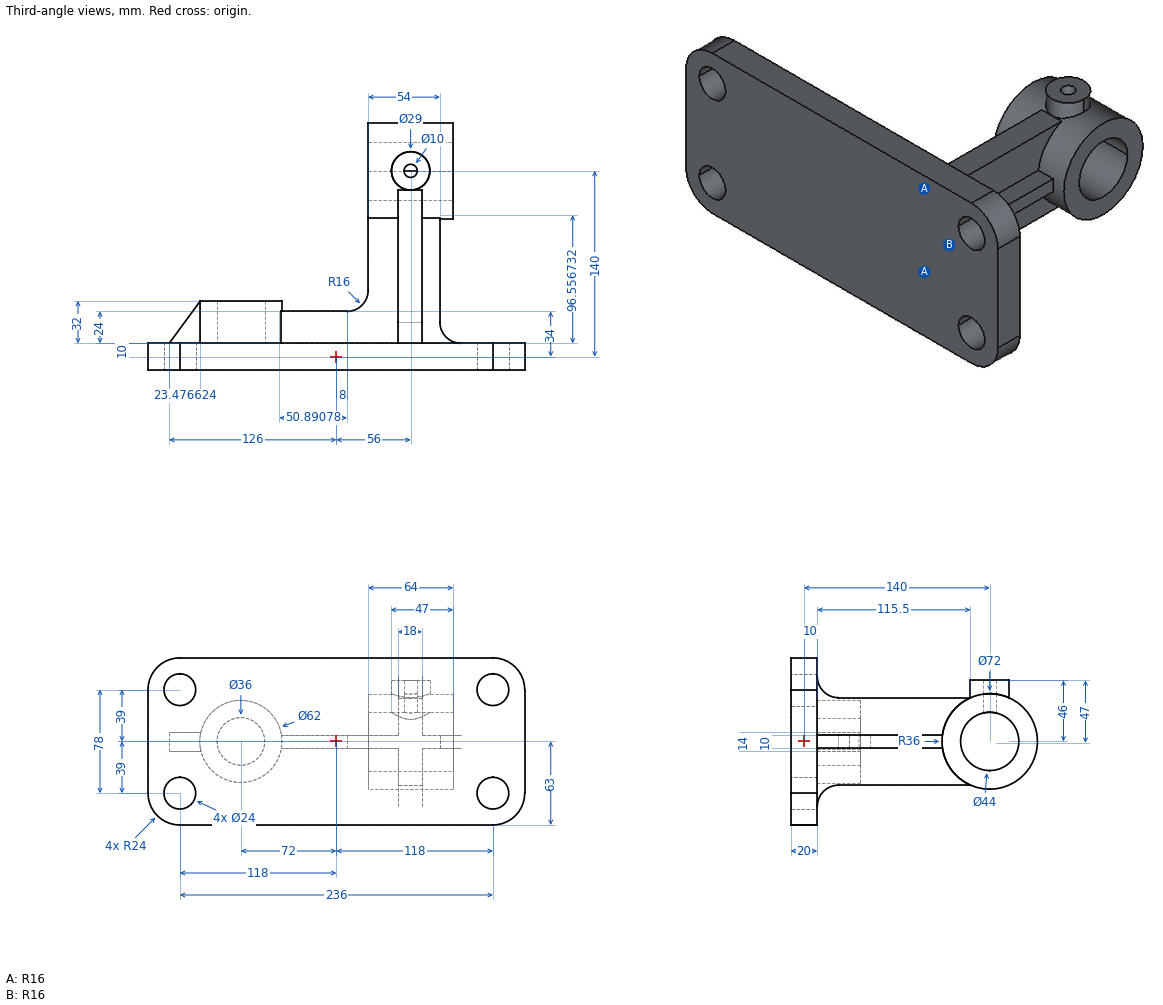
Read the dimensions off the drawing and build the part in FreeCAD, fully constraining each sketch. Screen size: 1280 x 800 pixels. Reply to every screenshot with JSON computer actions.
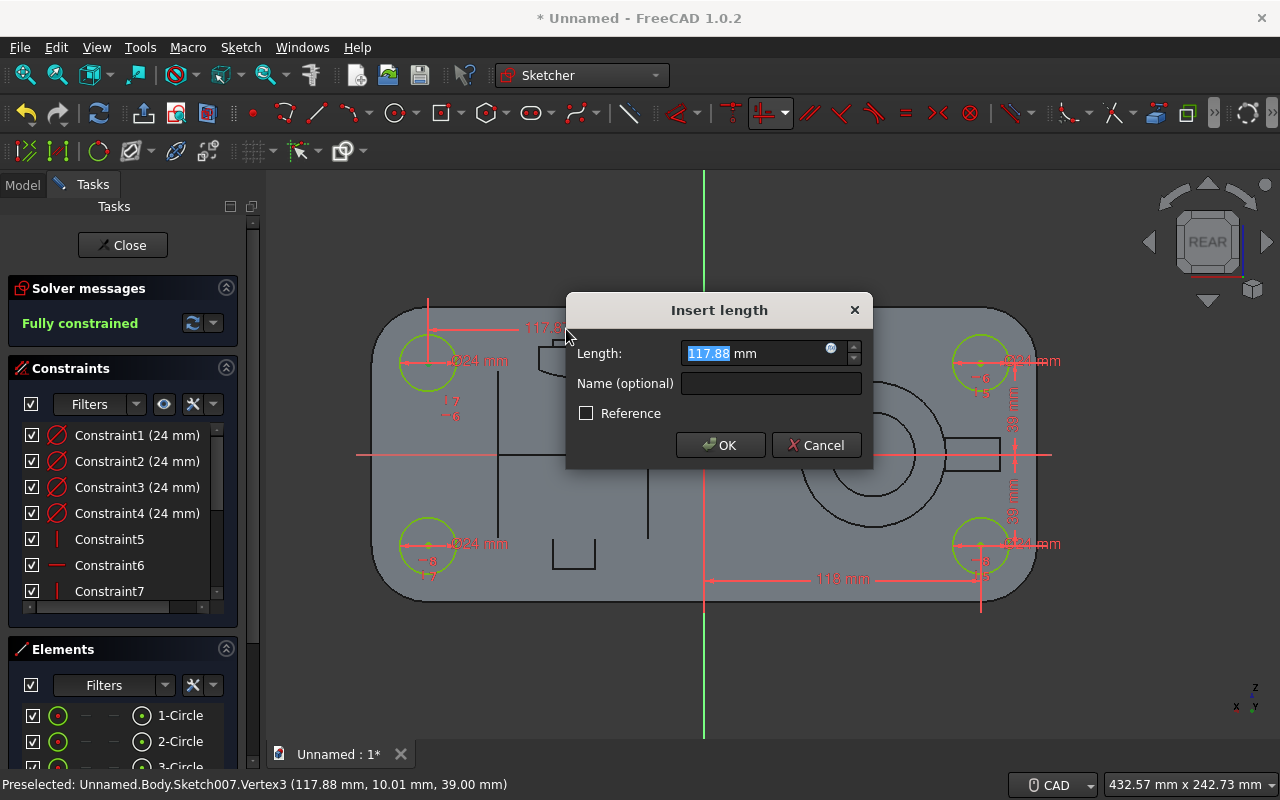
{"action": "type", "text": "118"}
{"action": "key", "text": "Return"}
{"action": "key", "text": "Escape"}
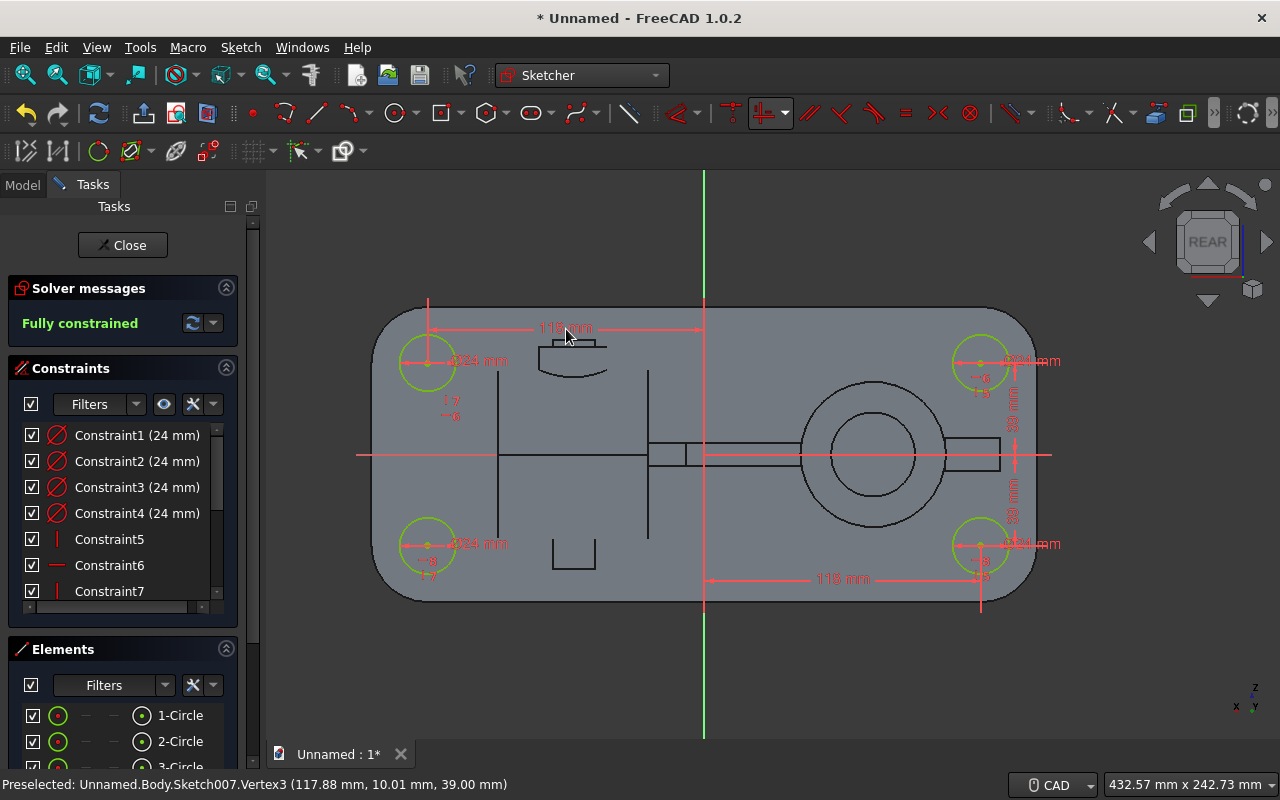
{"action": "left_click", "coordinate": [123, 245]}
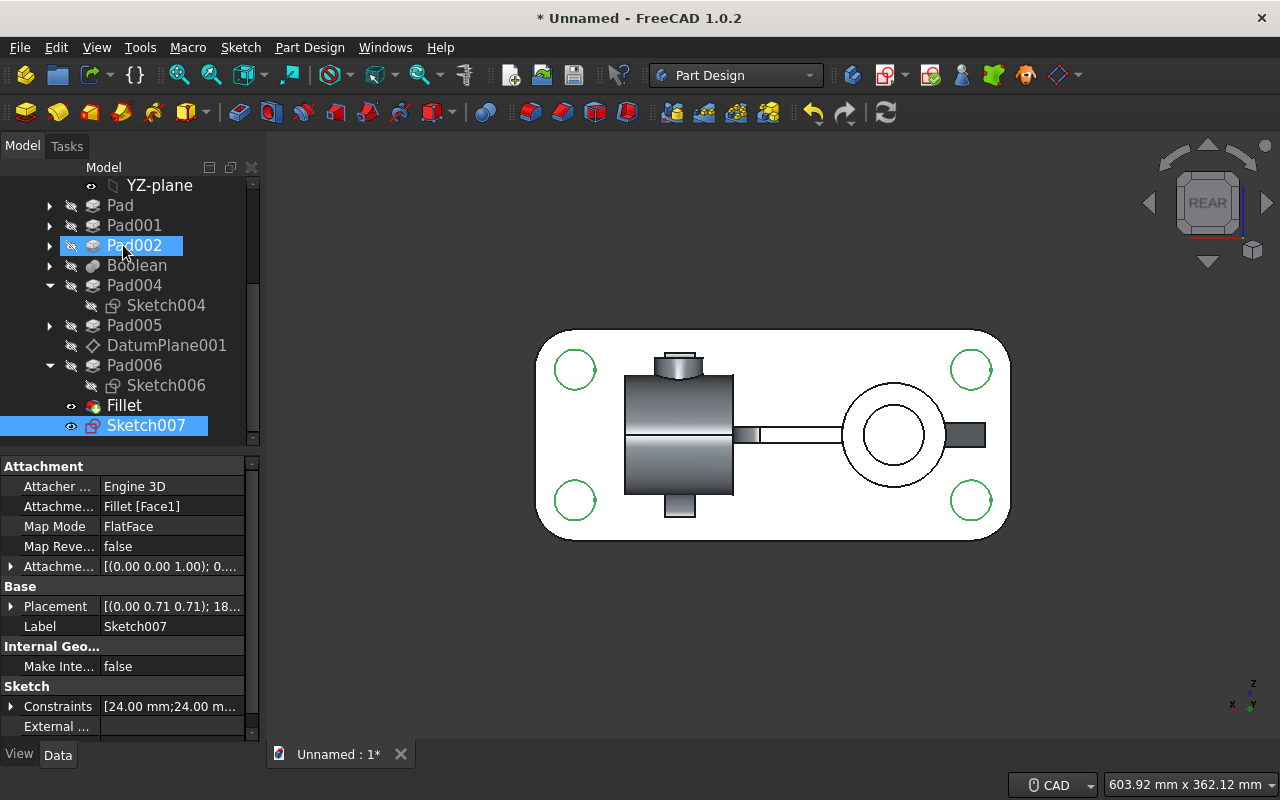
{"action": "left_click", "coordinate": [240, 112]}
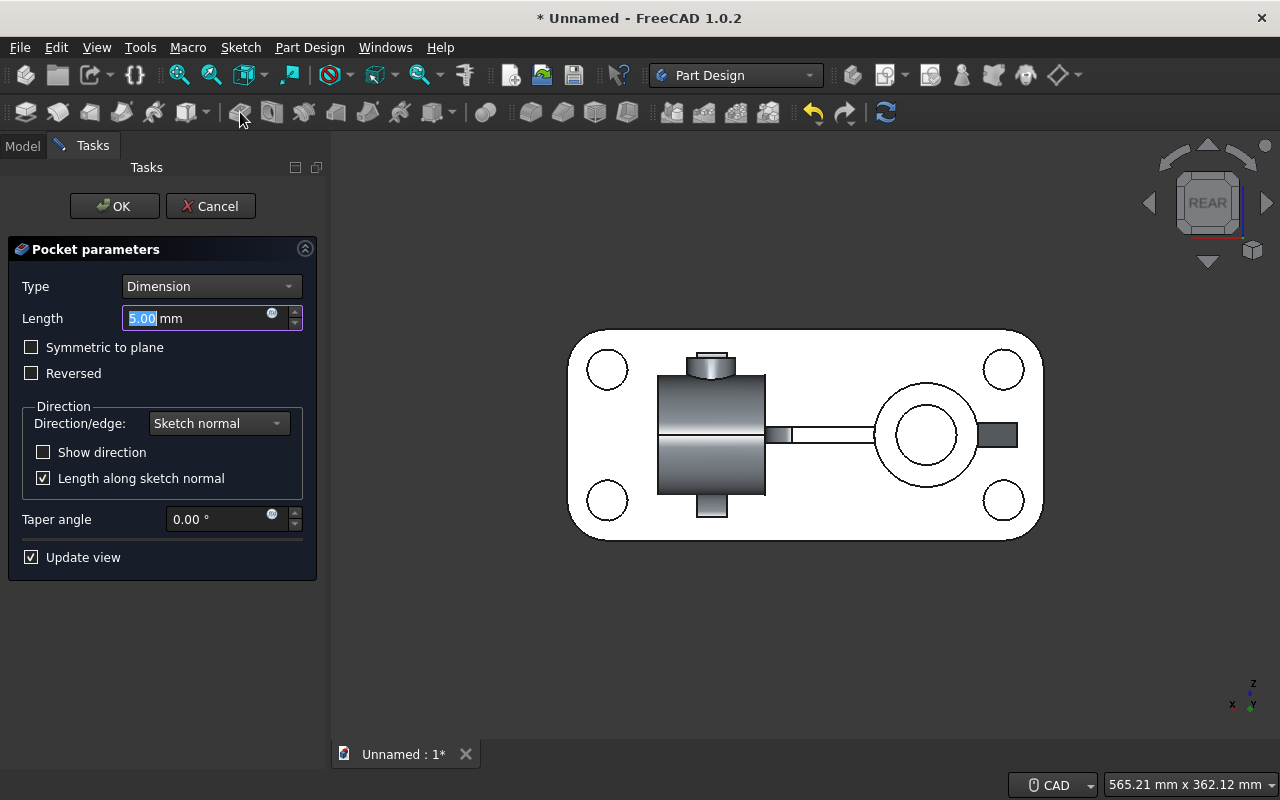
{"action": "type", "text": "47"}
{"action": "key", "text": "Tab"}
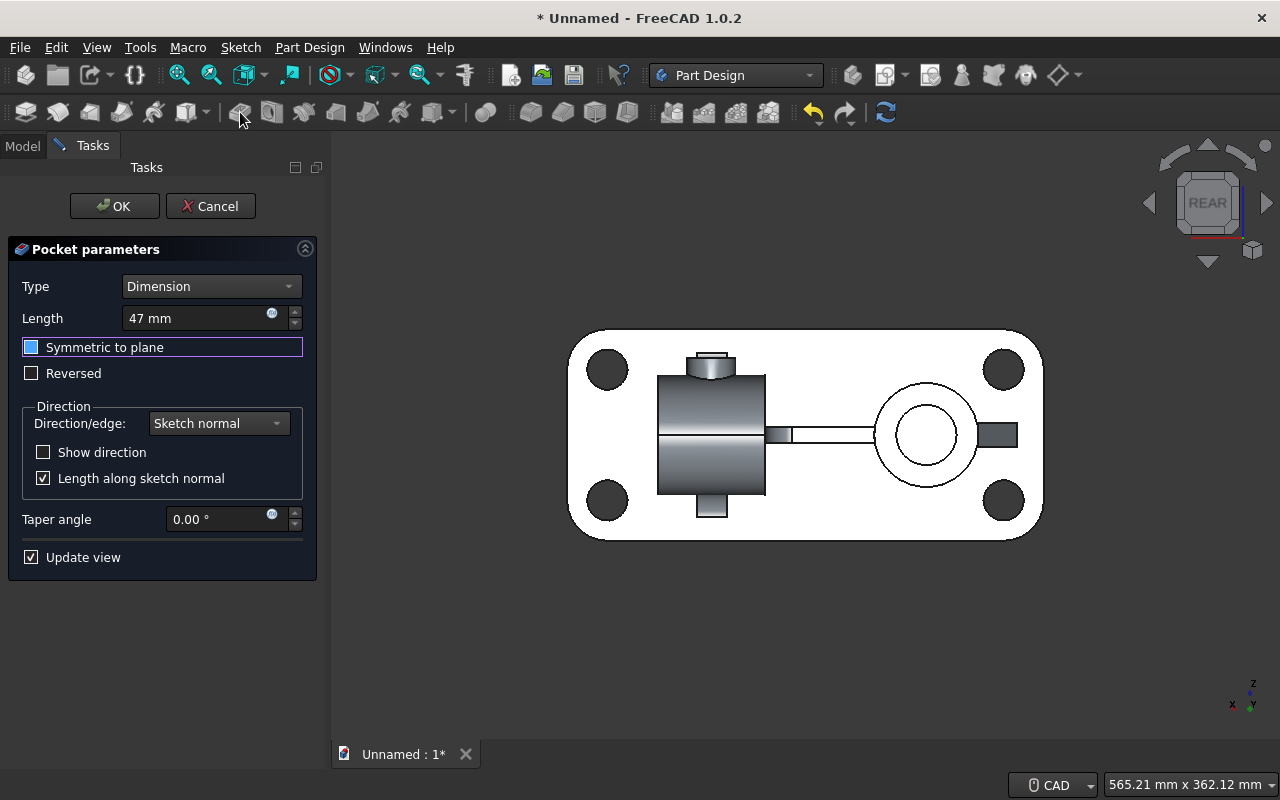
{"action": "left_click", "coordinate": [115, 206]}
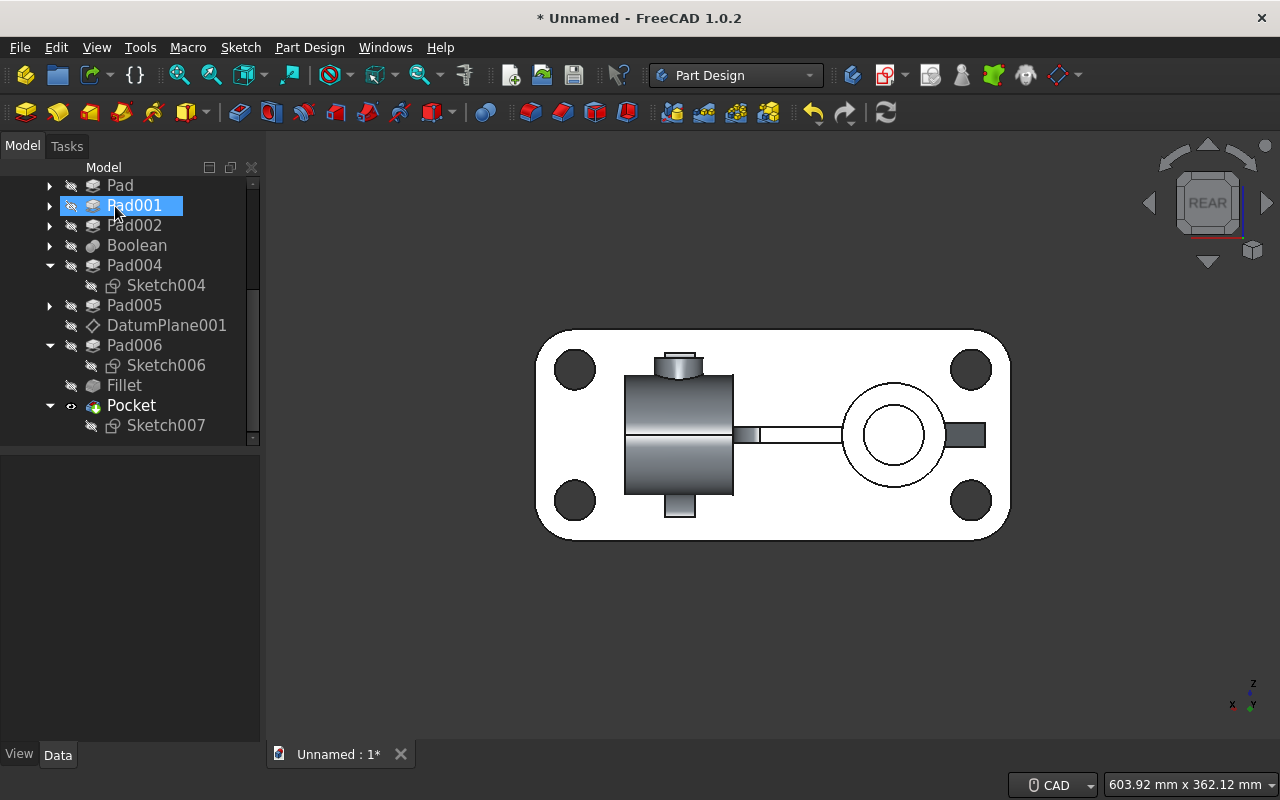
{"action": "key", "text": "0"}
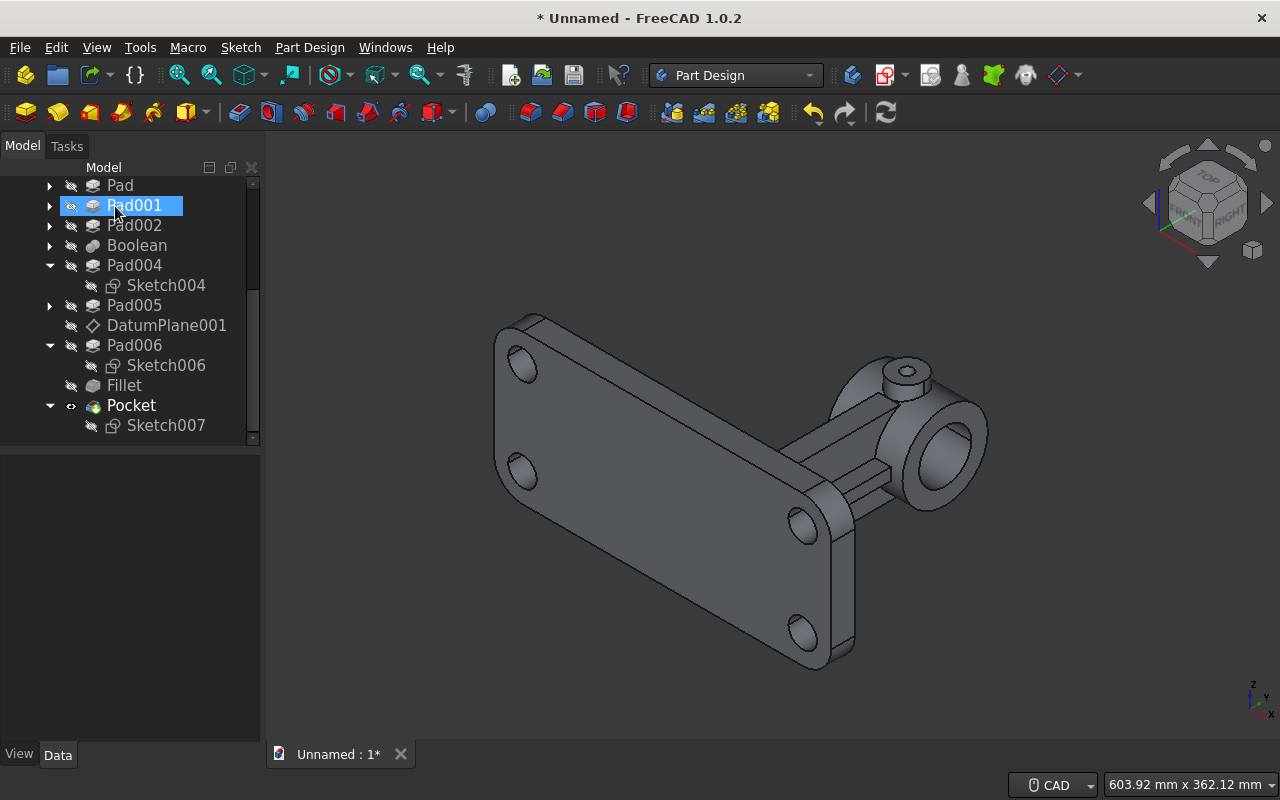
{"action": "left_click", "coordinate": [921, 498]}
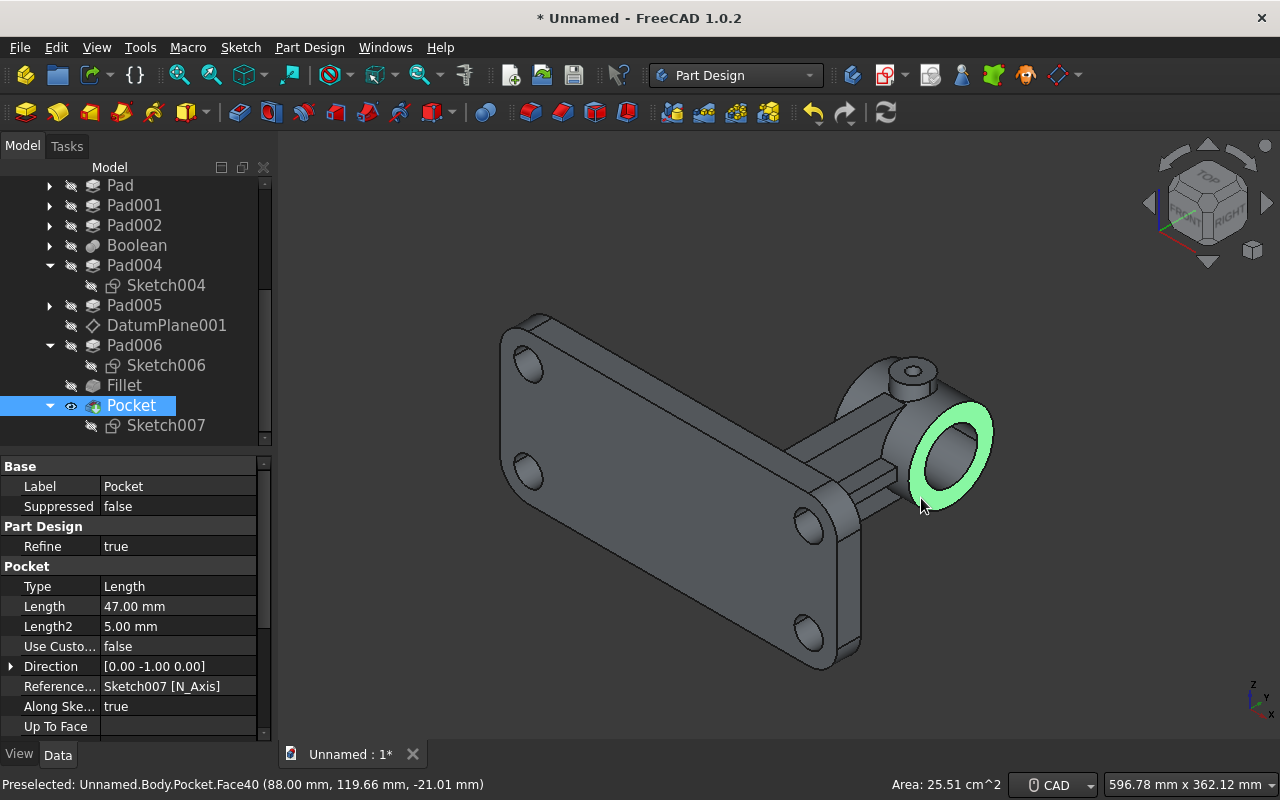
{"action": "left_click", "coordinate": [886, 76]}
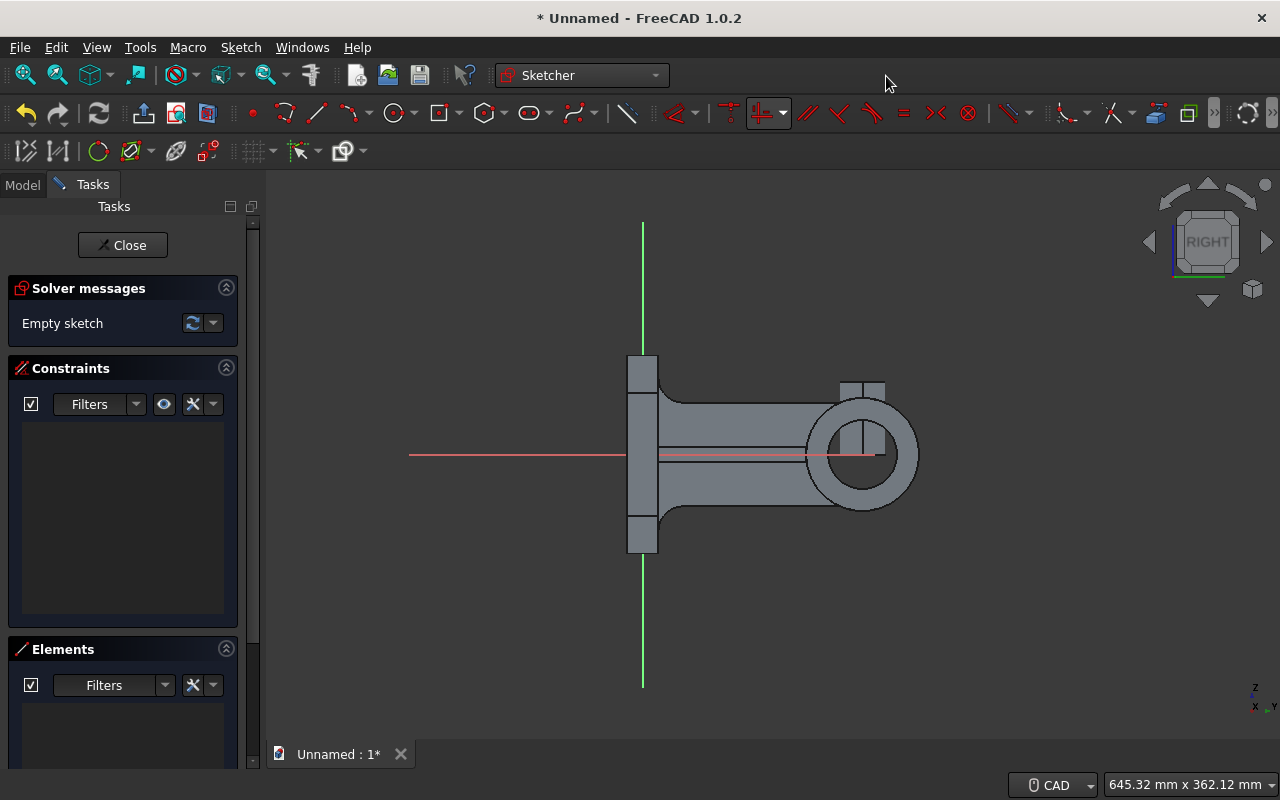
{"action": "left_click", "coordinate": [208, 114]}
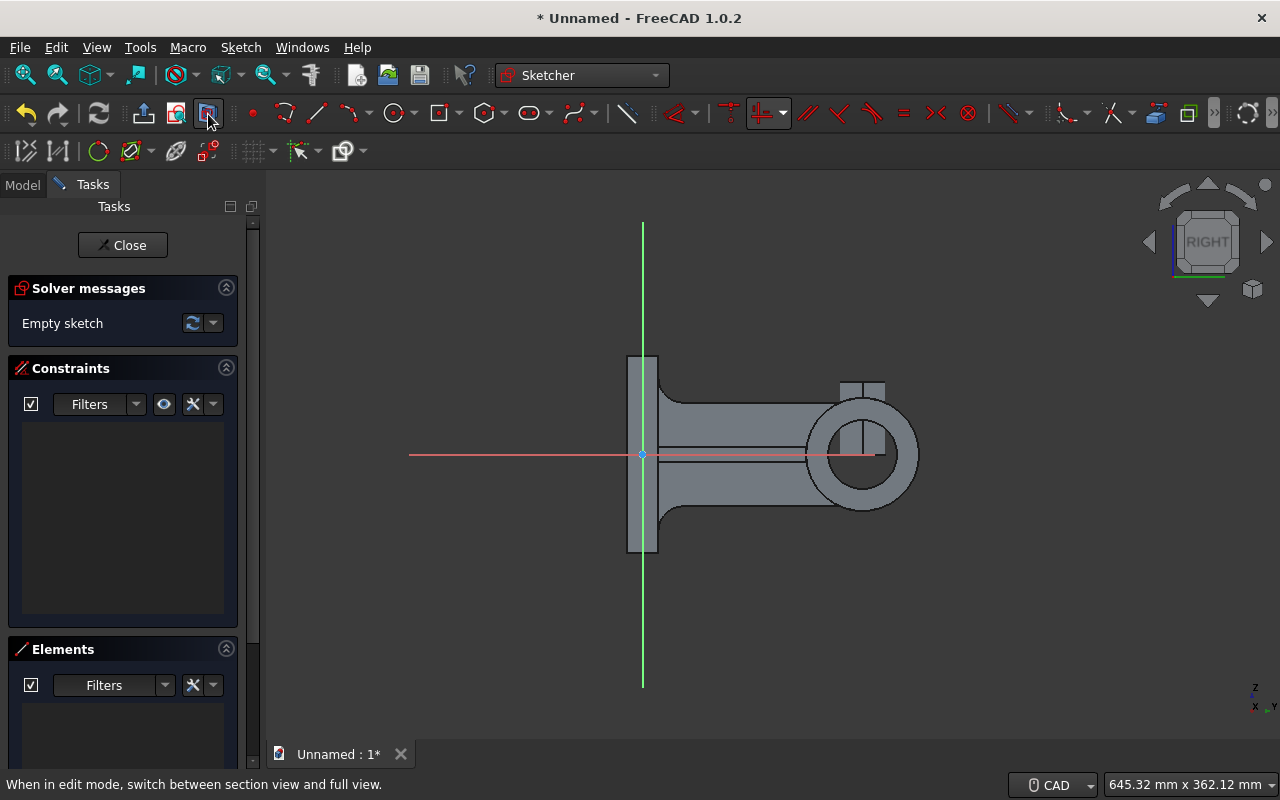
{"action": "scroll", "coordinate": [903, 455], "scroll_direction": "up", "scroll_amount": 8}